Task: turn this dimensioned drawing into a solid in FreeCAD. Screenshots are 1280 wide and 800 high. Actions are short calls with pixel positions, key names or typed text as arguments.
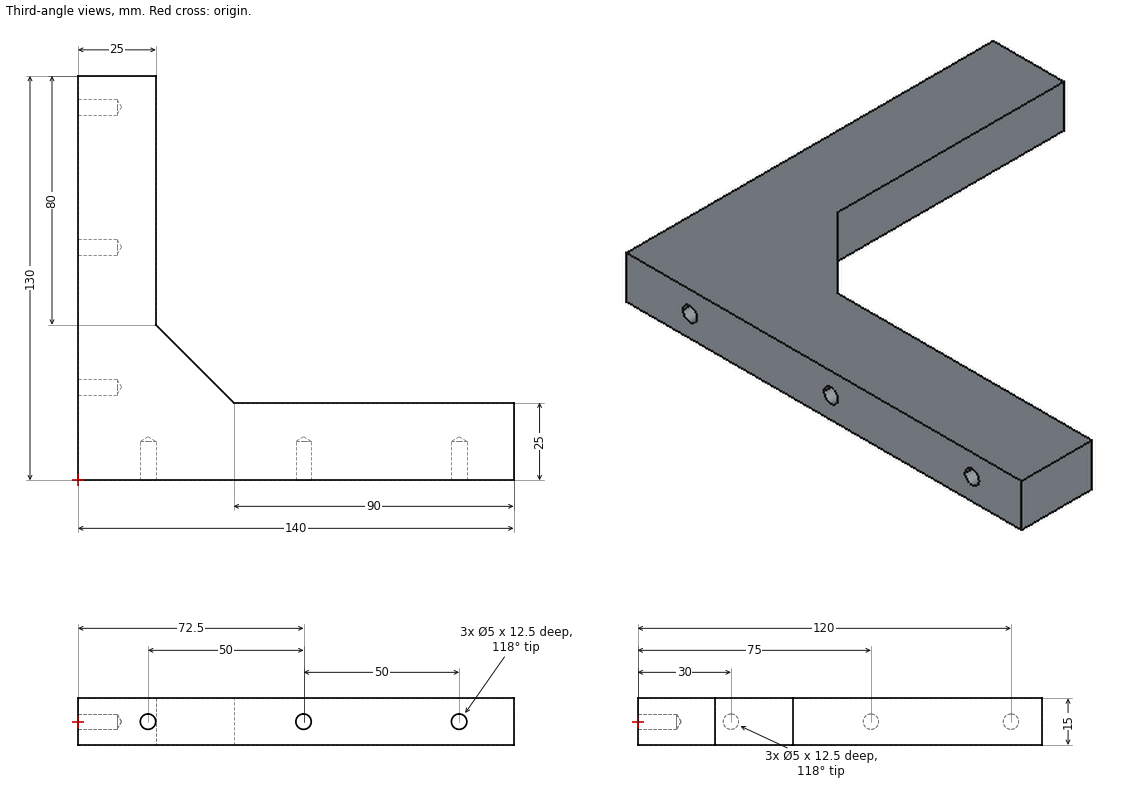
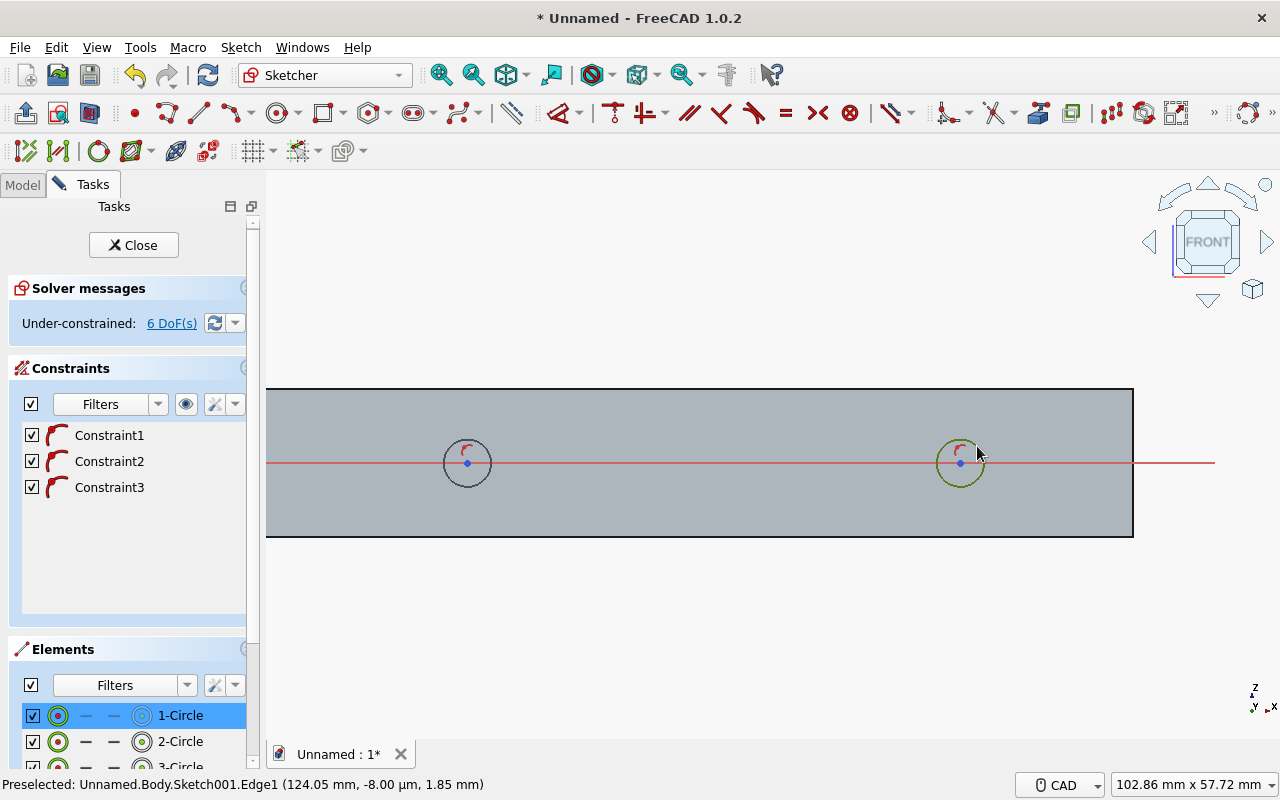
click(484, 446)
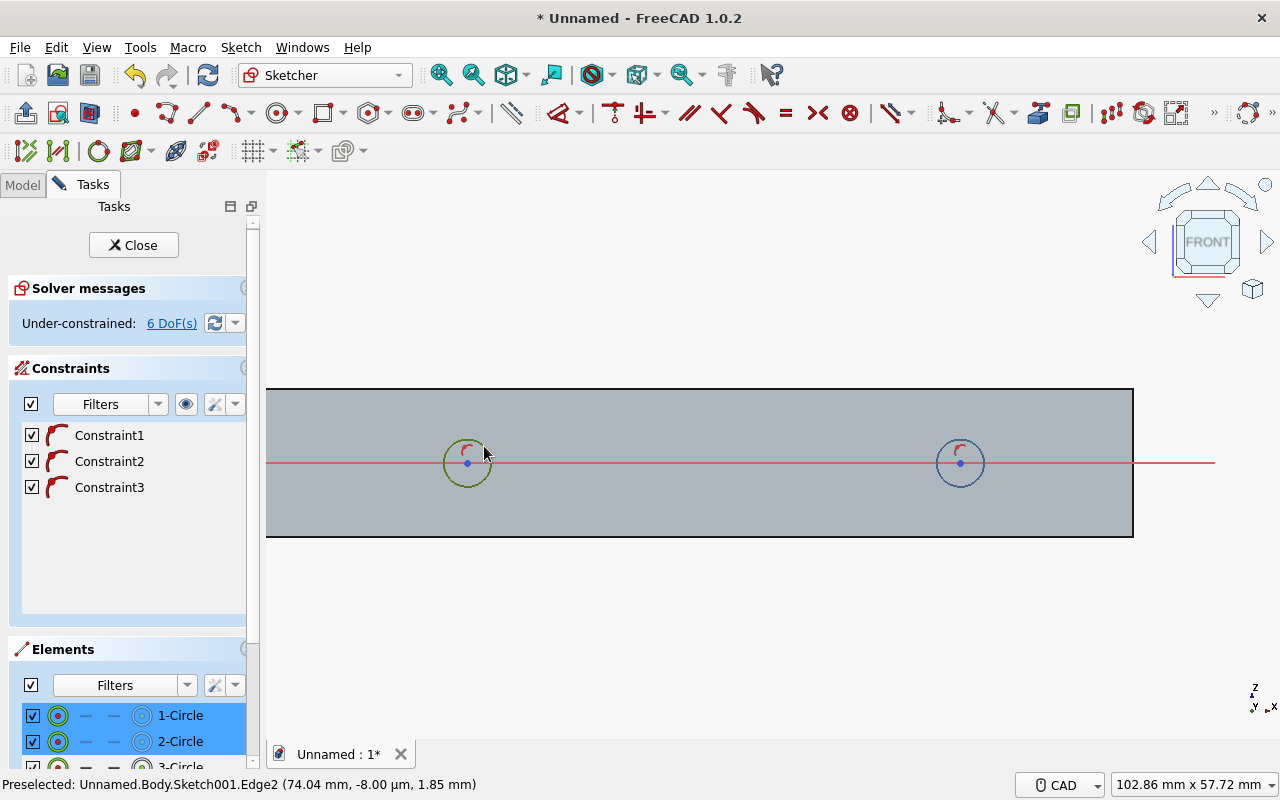
scroll(978, 447, down, 4)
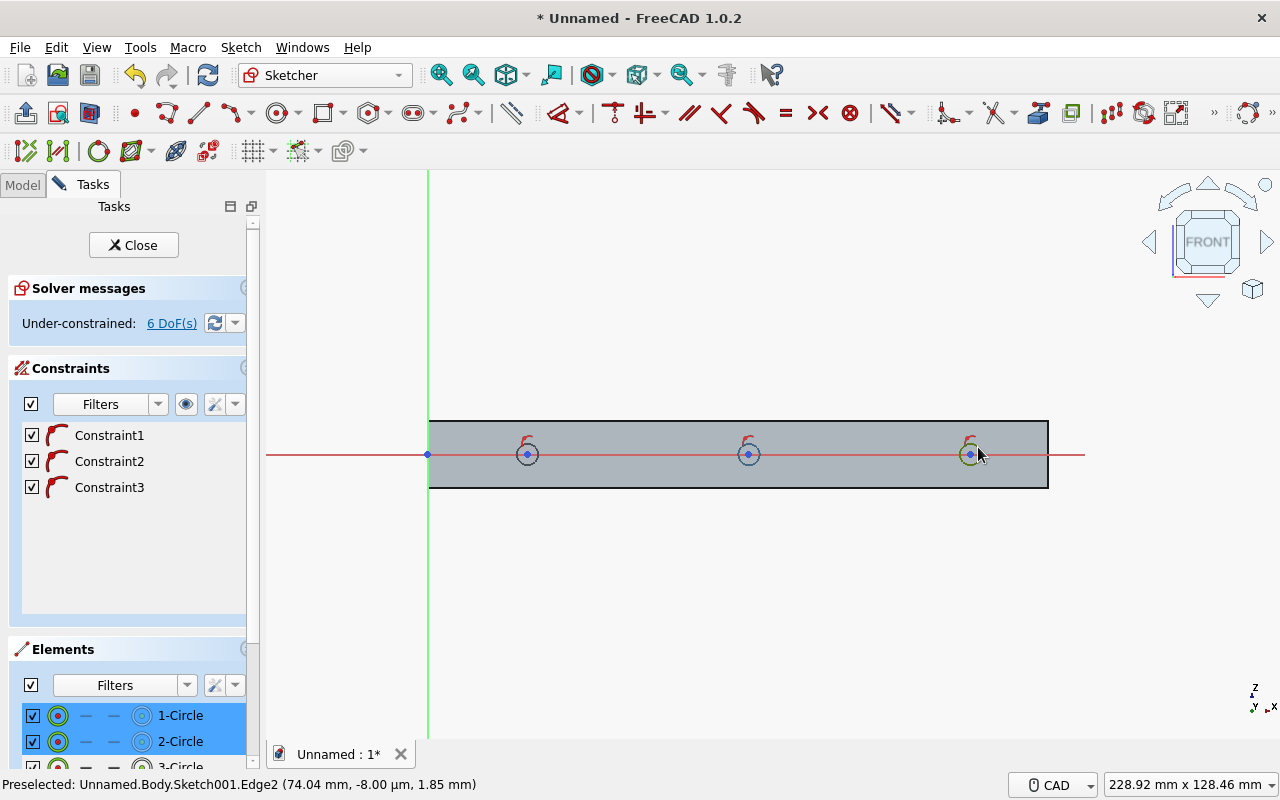
scroll(535, 447, up, 4)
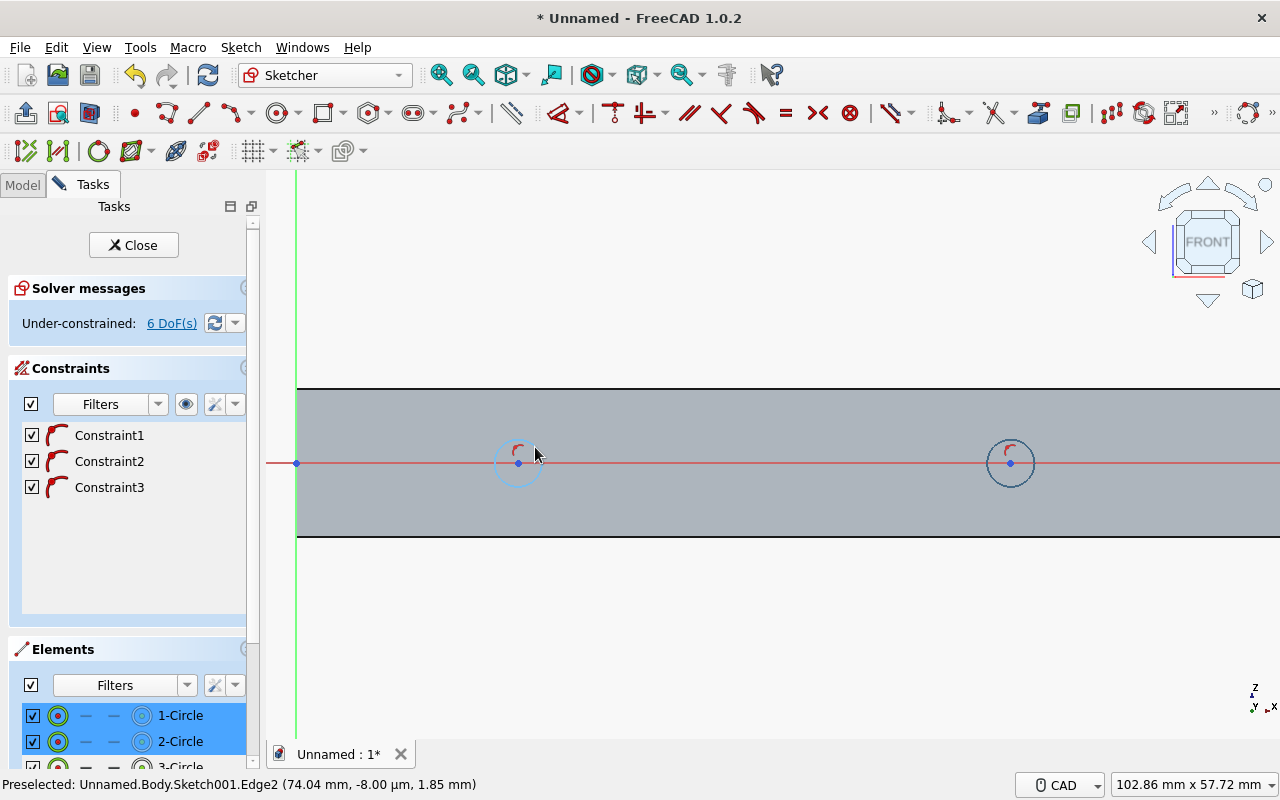
click(535, 446)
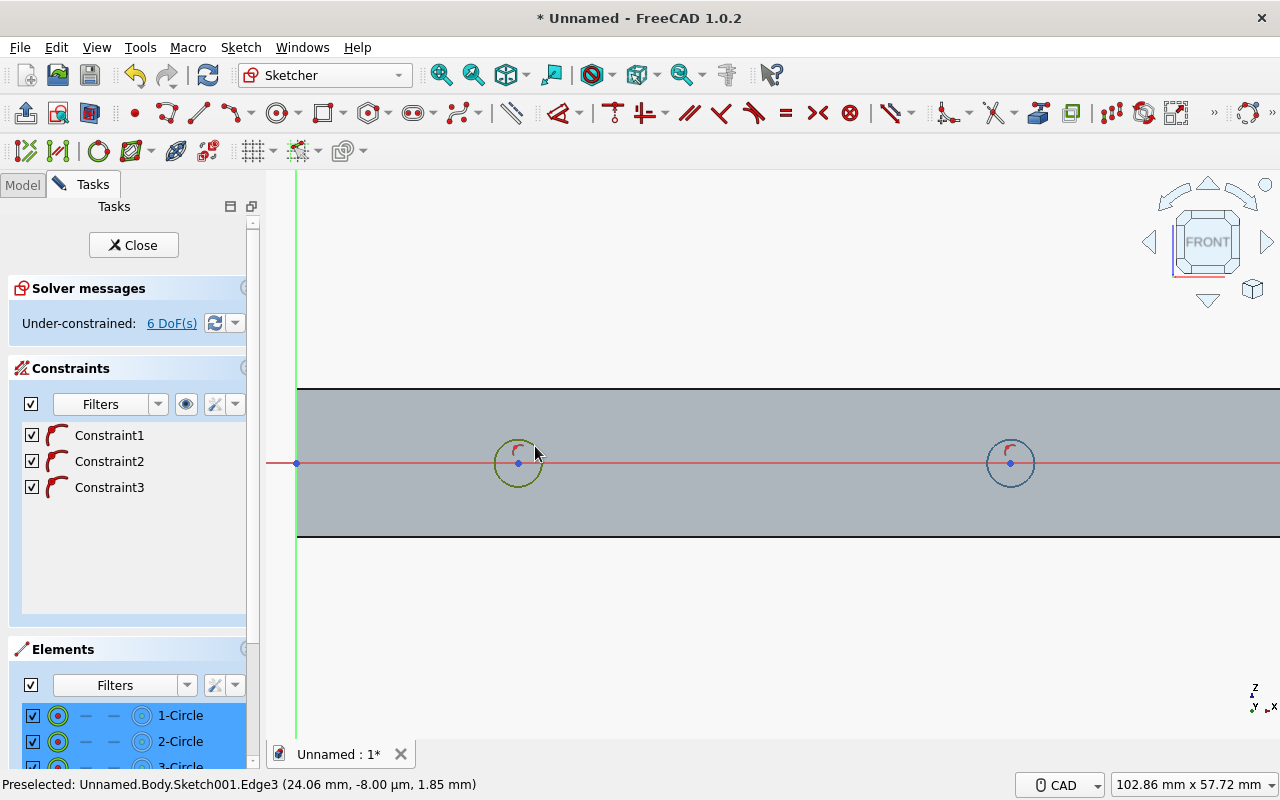
click(786, 114)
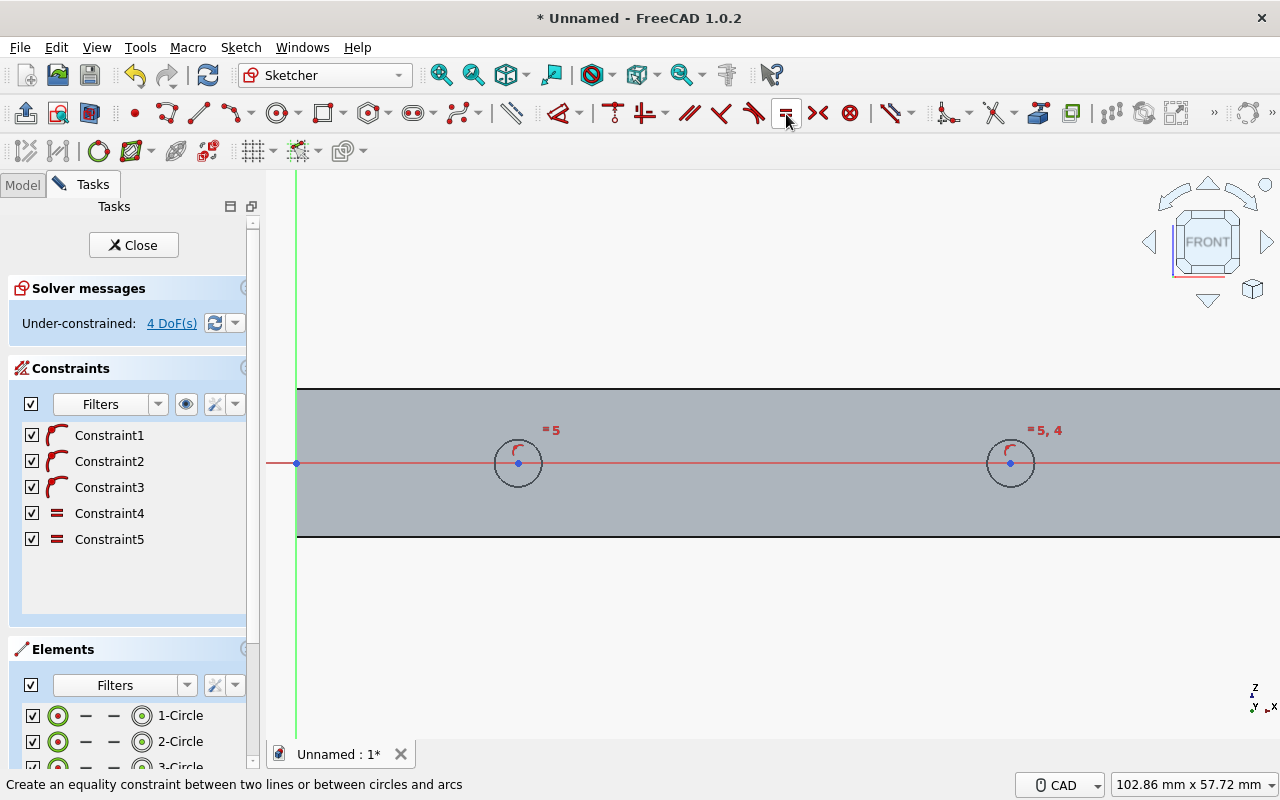
click(558, 114)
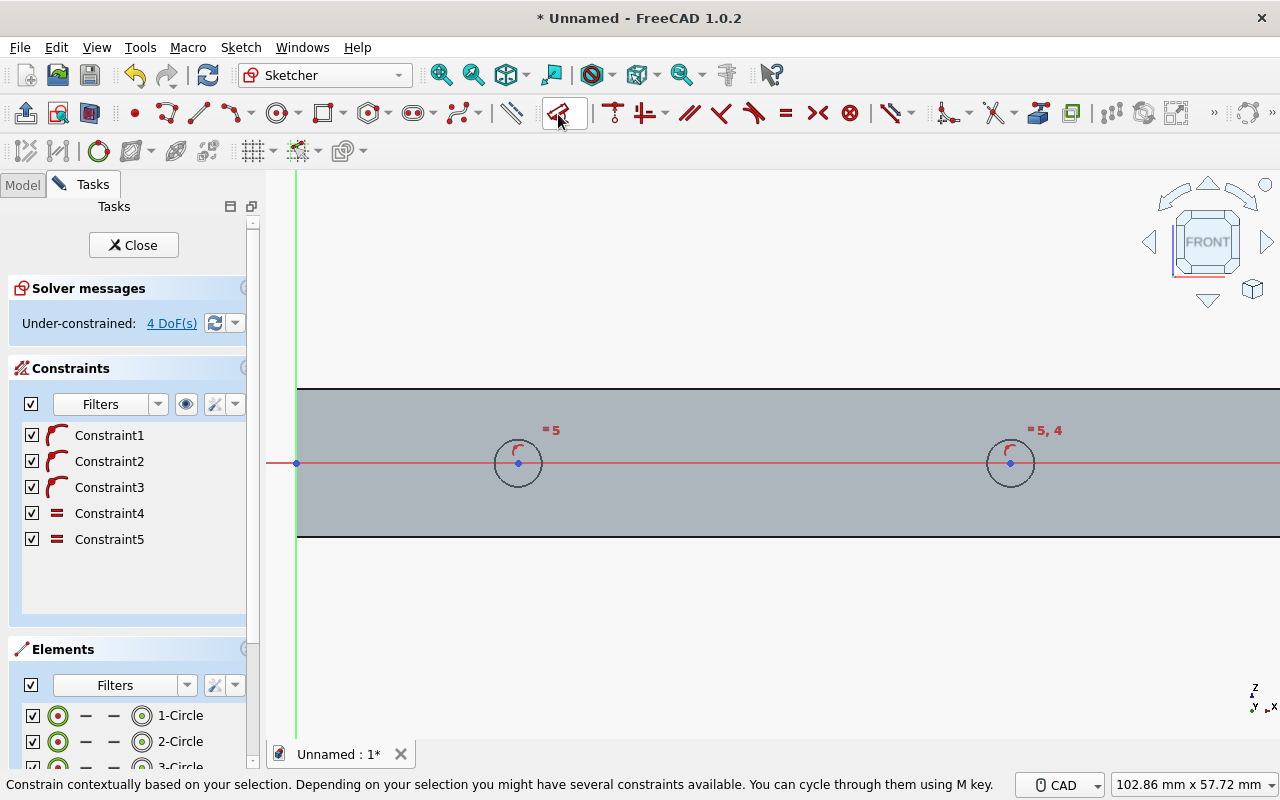
scroll(535, 447, down, 4)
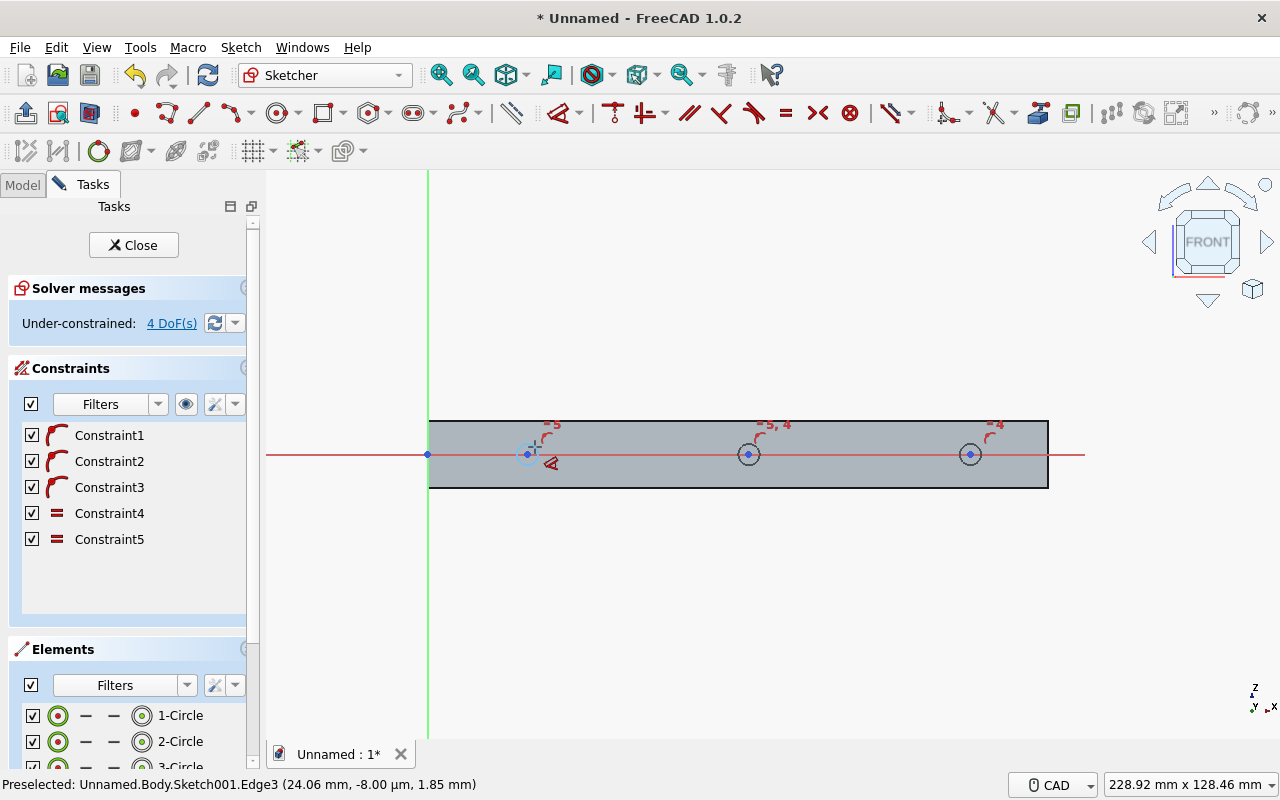
scroll(978, 447, up, 4)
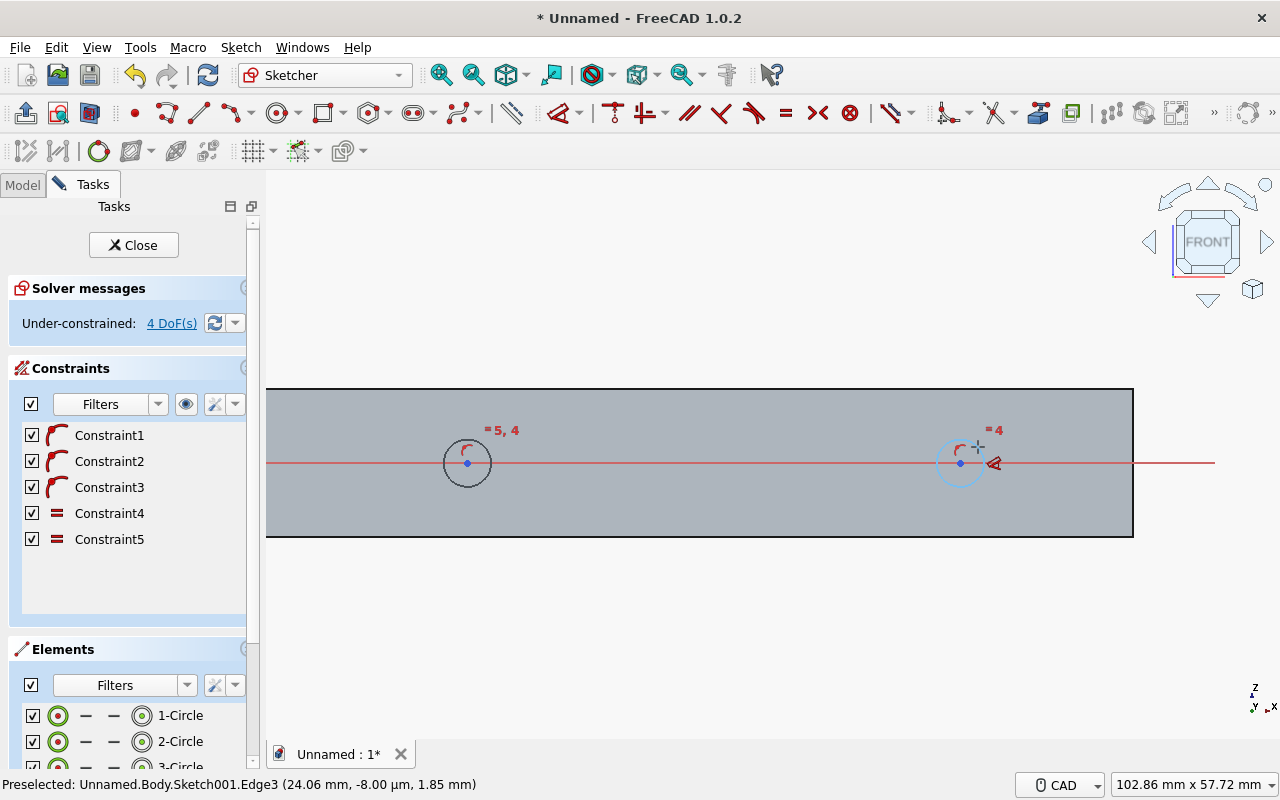
click(977, 446)
click(999, 423)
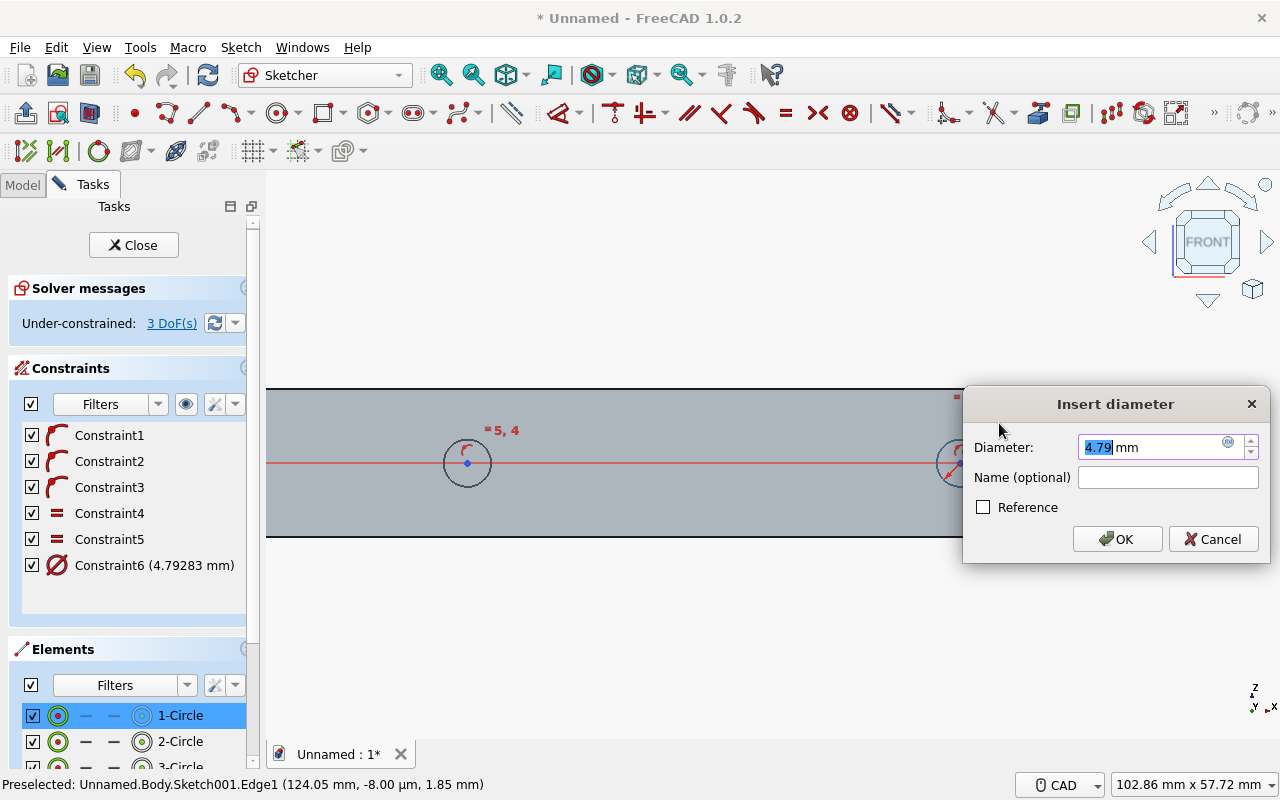
text(5)
key(Return)